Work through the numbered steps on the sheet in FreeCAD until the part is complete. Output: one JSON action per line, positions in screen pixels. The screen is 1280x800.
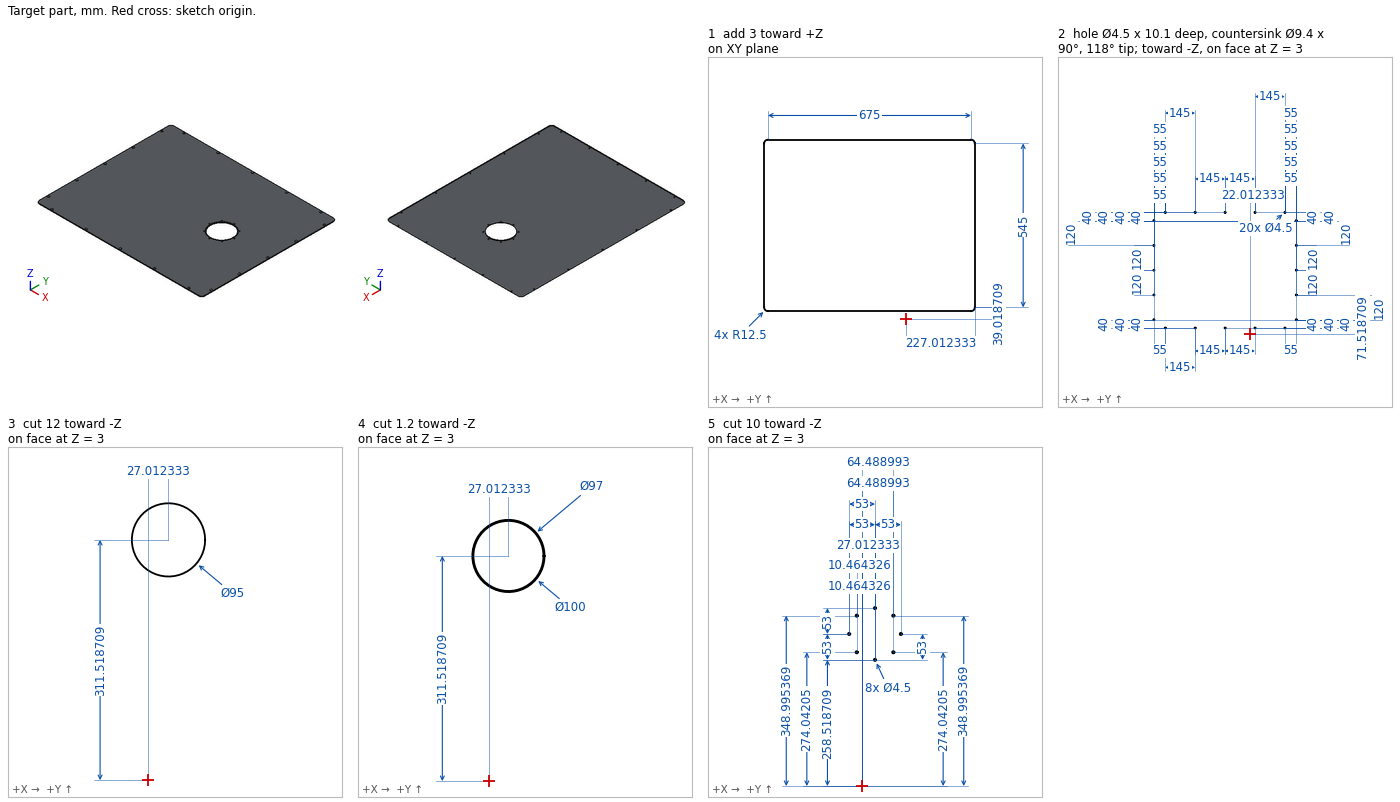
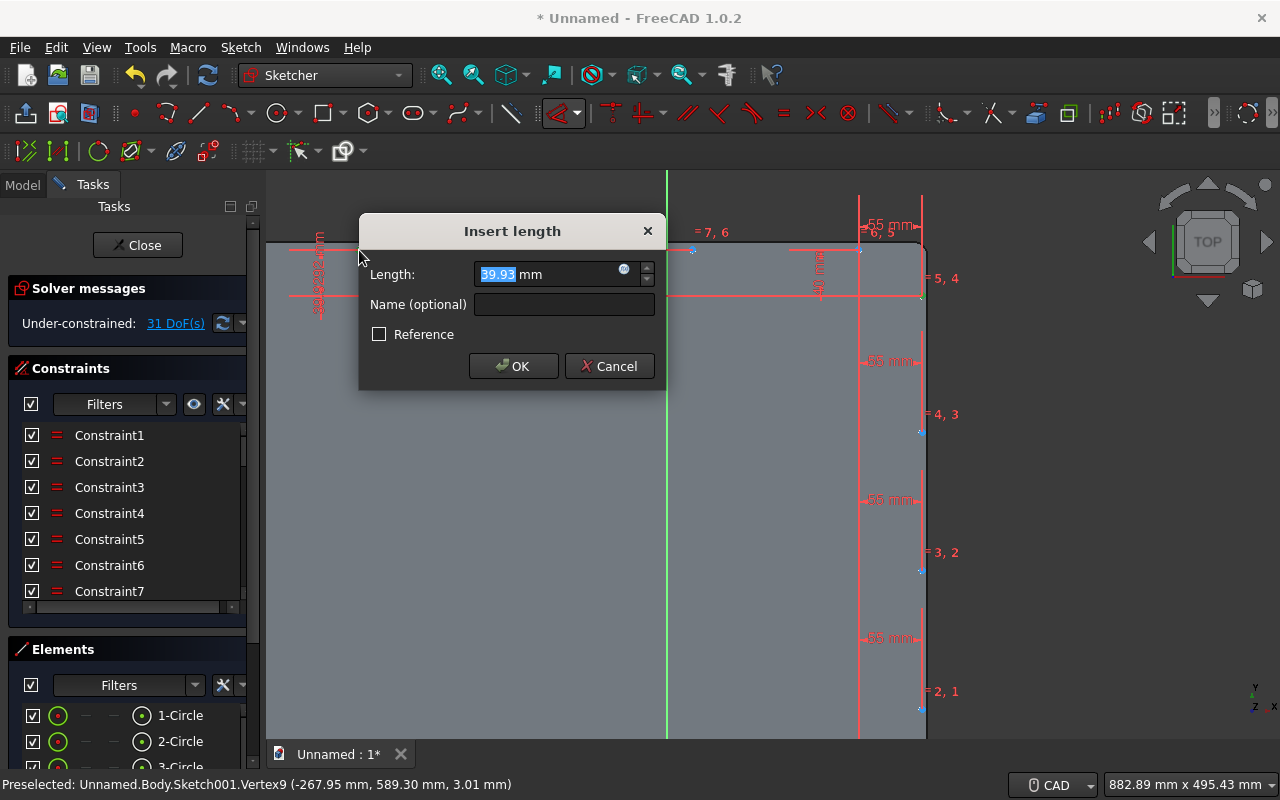
{"action": "type", "text": "40"}
{"action": "key", "text": "Return"}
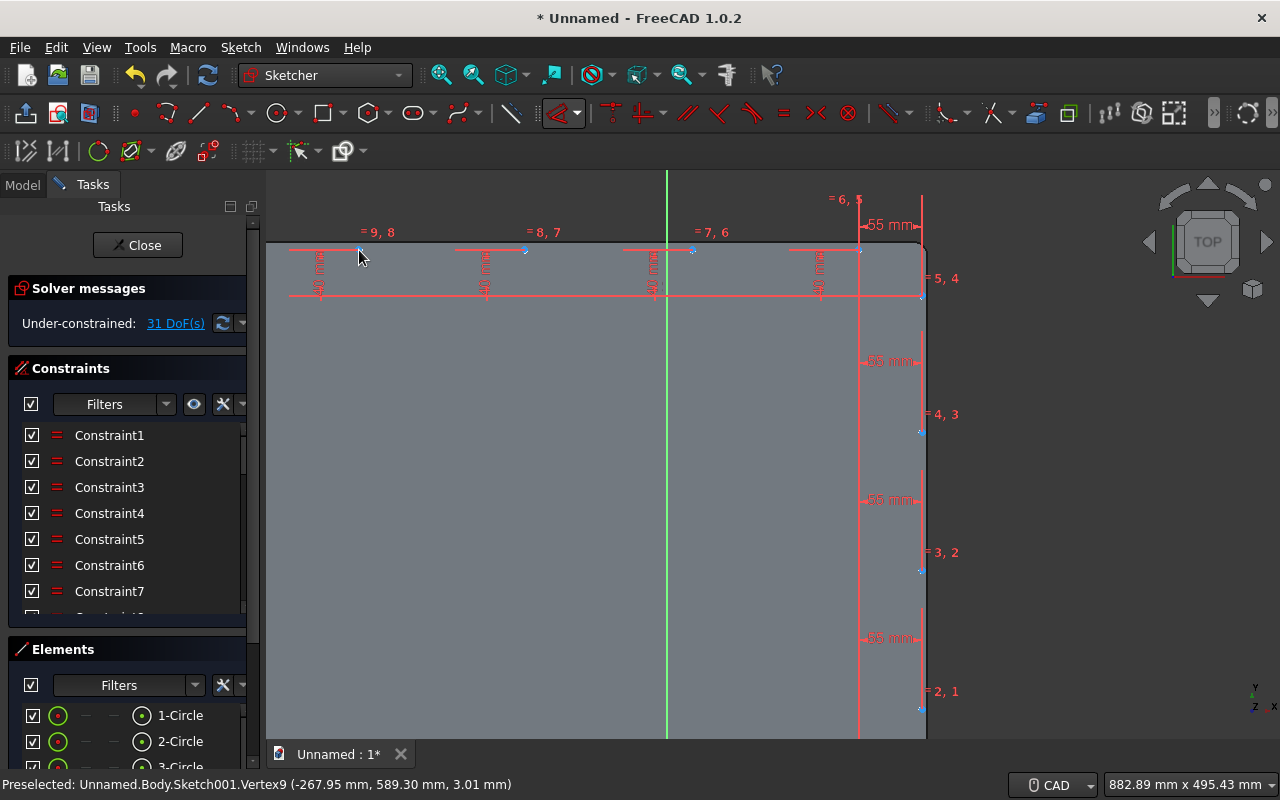
{"action": "left_click", "coordinate": [922, 296]}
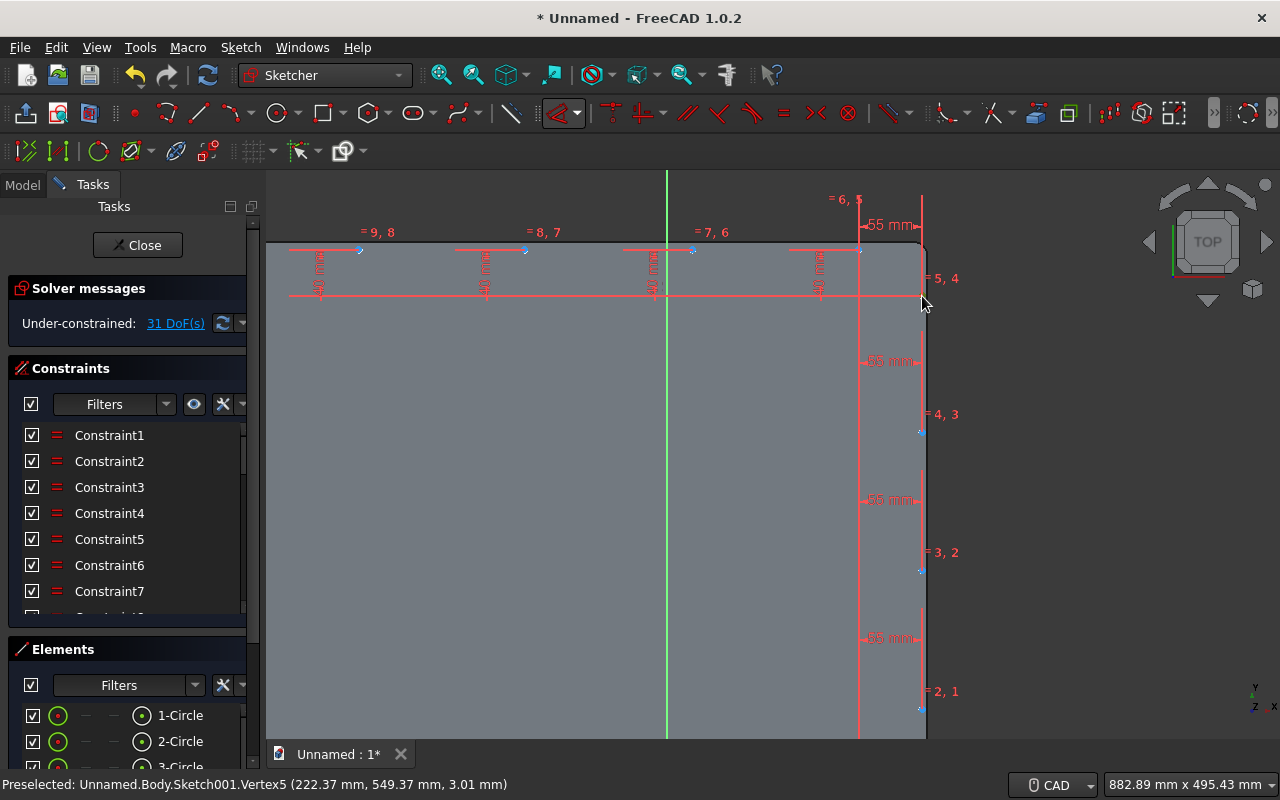
{"action": "scroll", "coordinate": [922, 295], "scroll_direction": "down", "scroll_amount": 3}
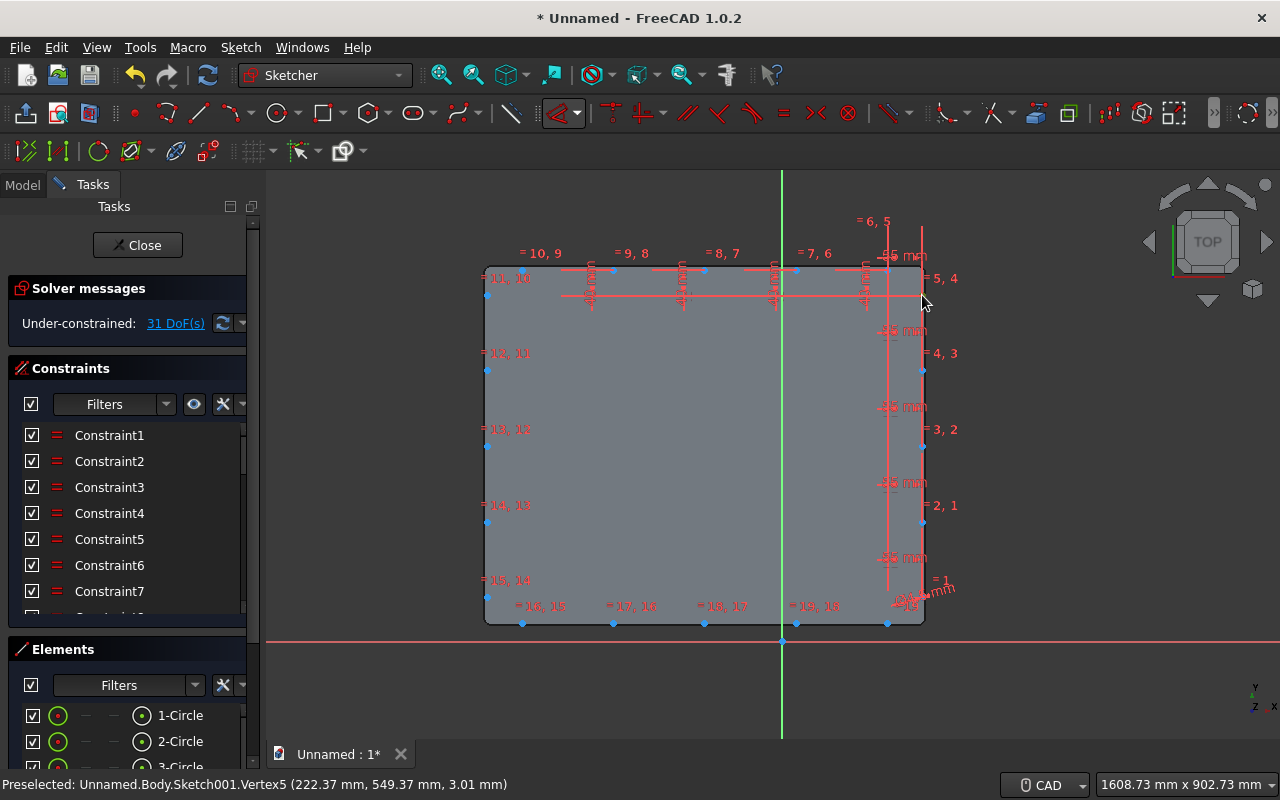
{"action": "scroll", "coordinate": [522, 270], "scroll_direction": "up", "scroll_amount": 3}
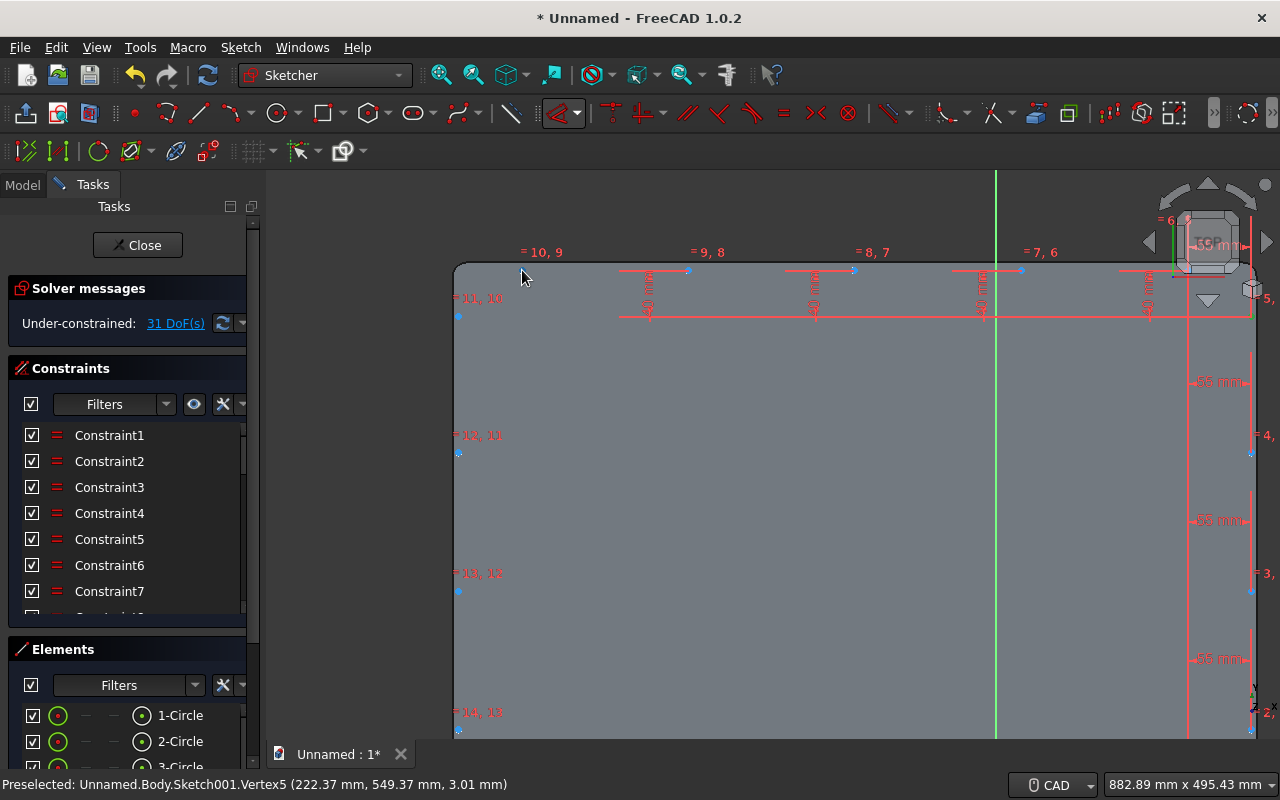
{"action": "left_click", "coordinate": [522, 271]}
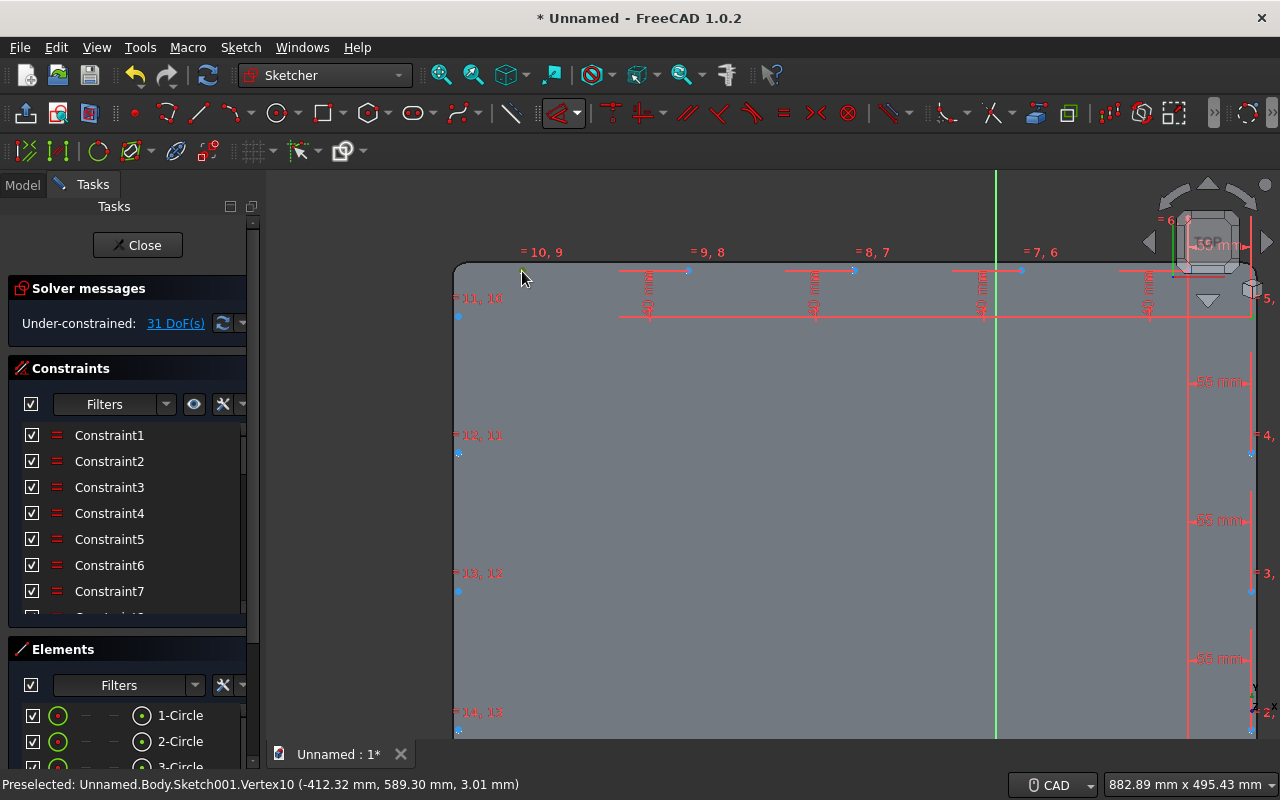
{"action": "left_click", "coordinate": [580, 114]}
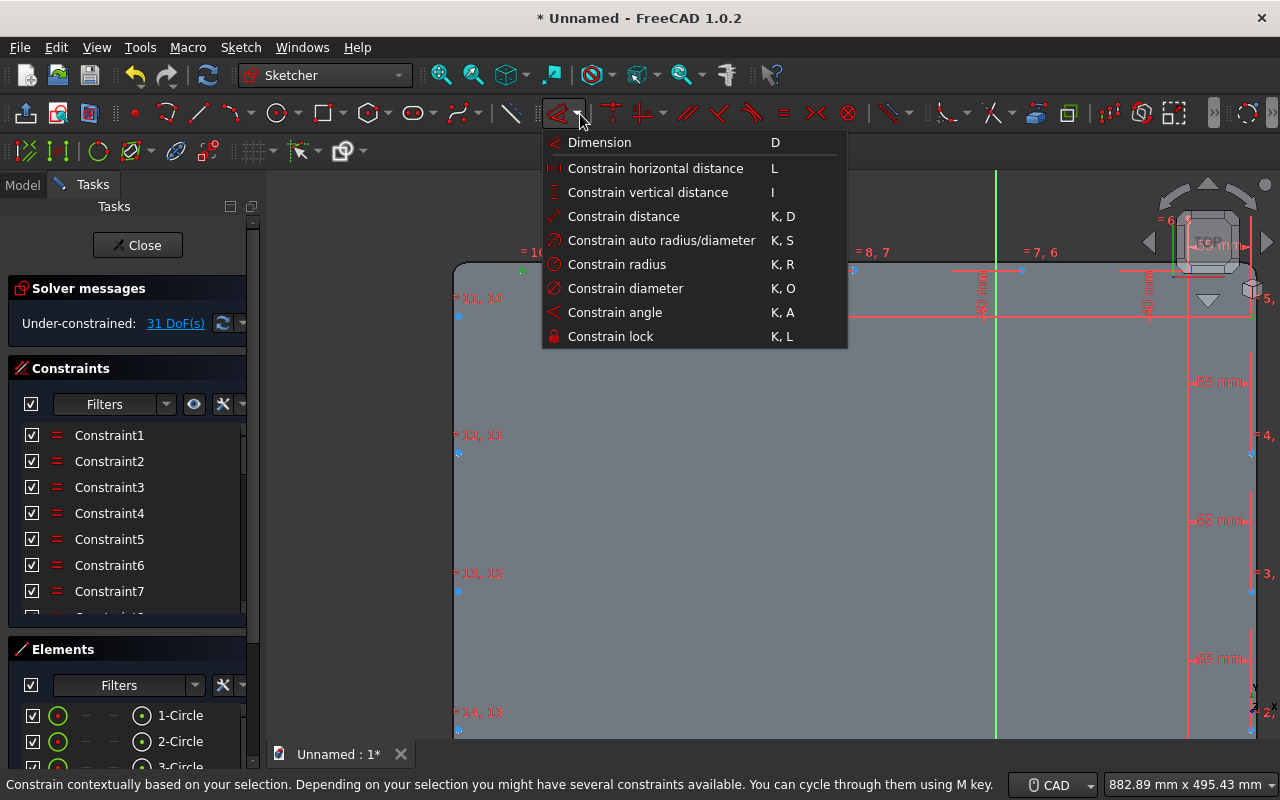
{"action": "left_click", "coordinate": [695, 192]}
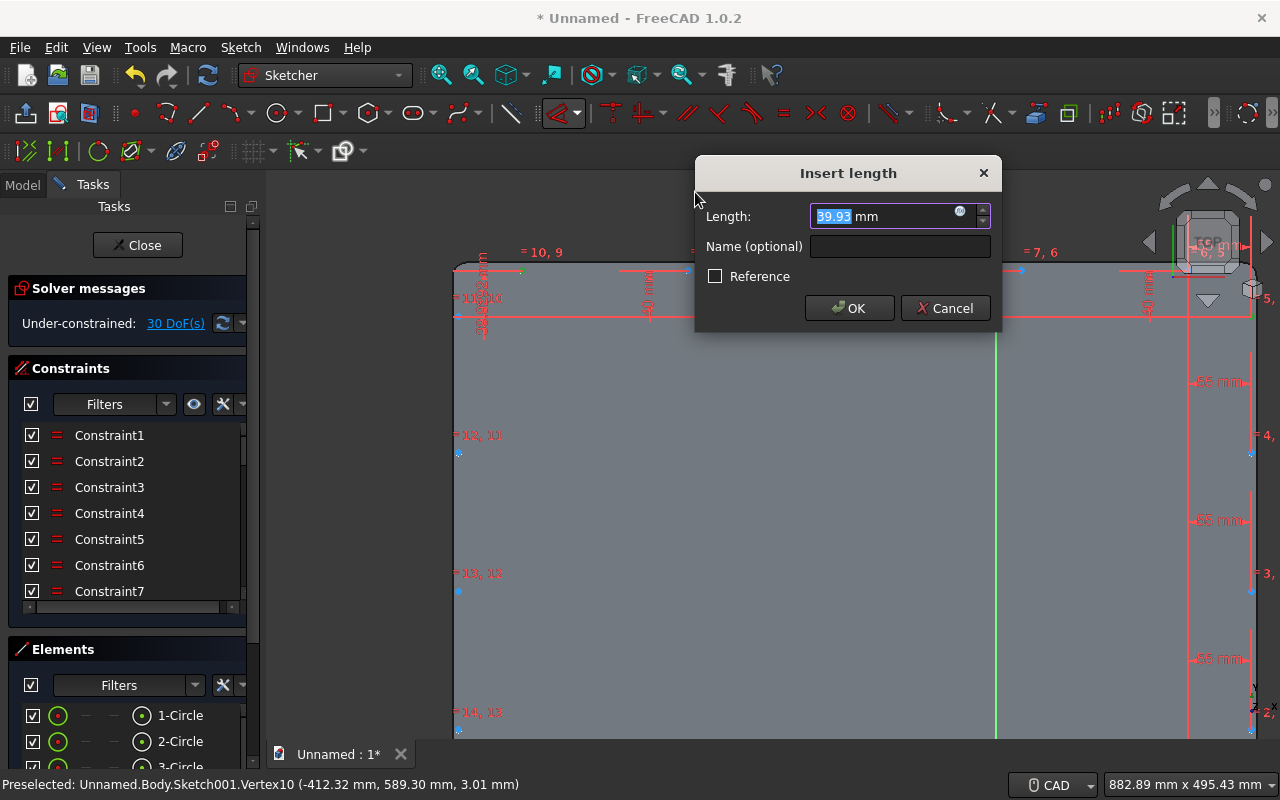
{"action": "type", "text": "40"}
{"action": "key", "text": "Return"}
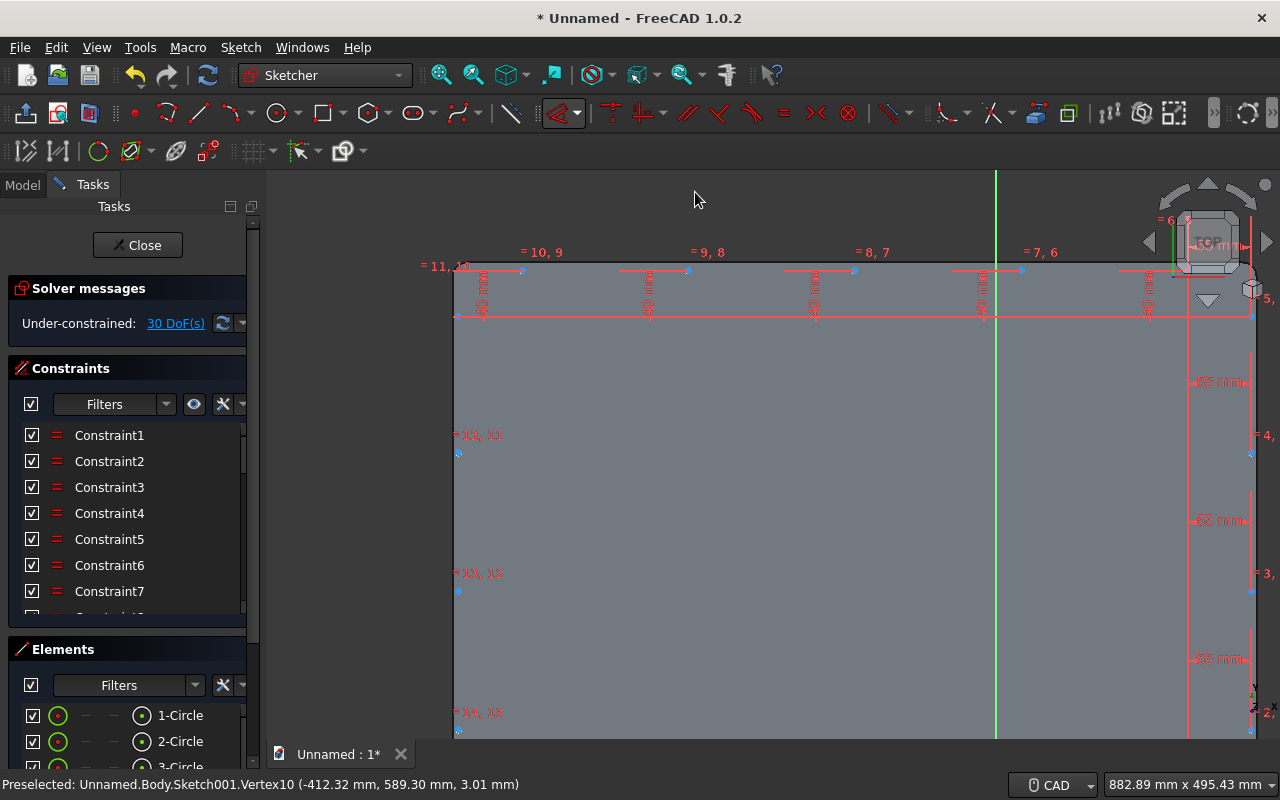
{"action": "left_click", "coordinate": [522, 271]}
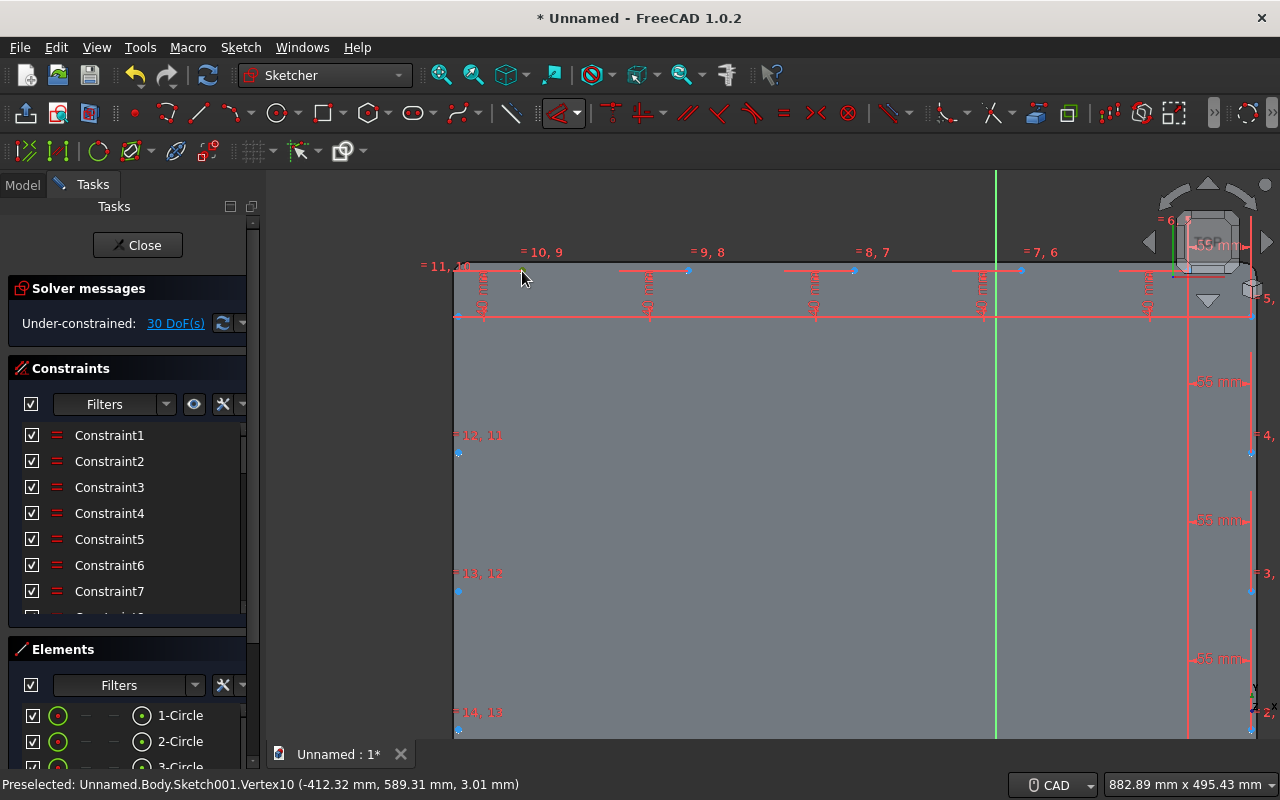
{"action": "left_click", "coordinate": [459, 316]}